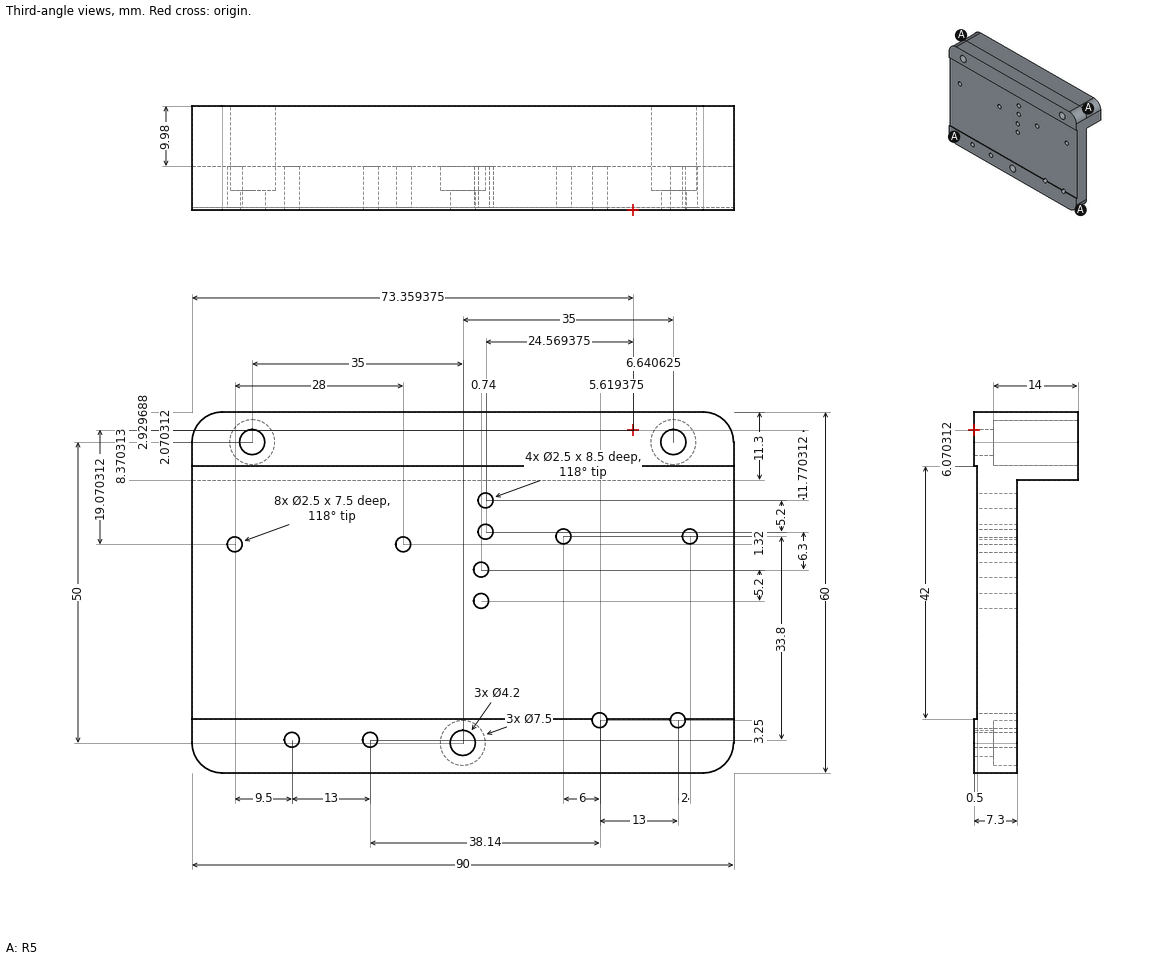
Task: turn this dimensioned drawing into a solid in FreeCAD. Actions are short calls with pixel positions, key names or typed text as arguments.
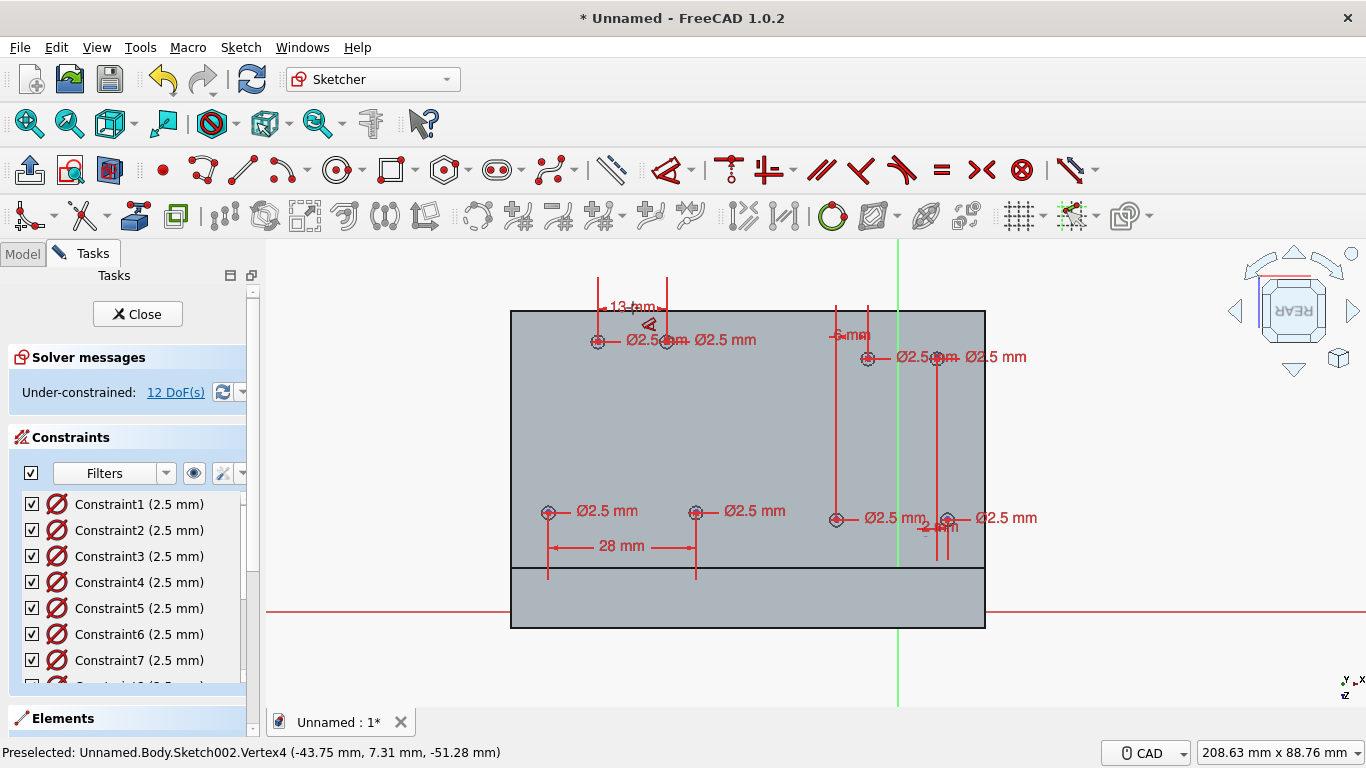
click(868, 359)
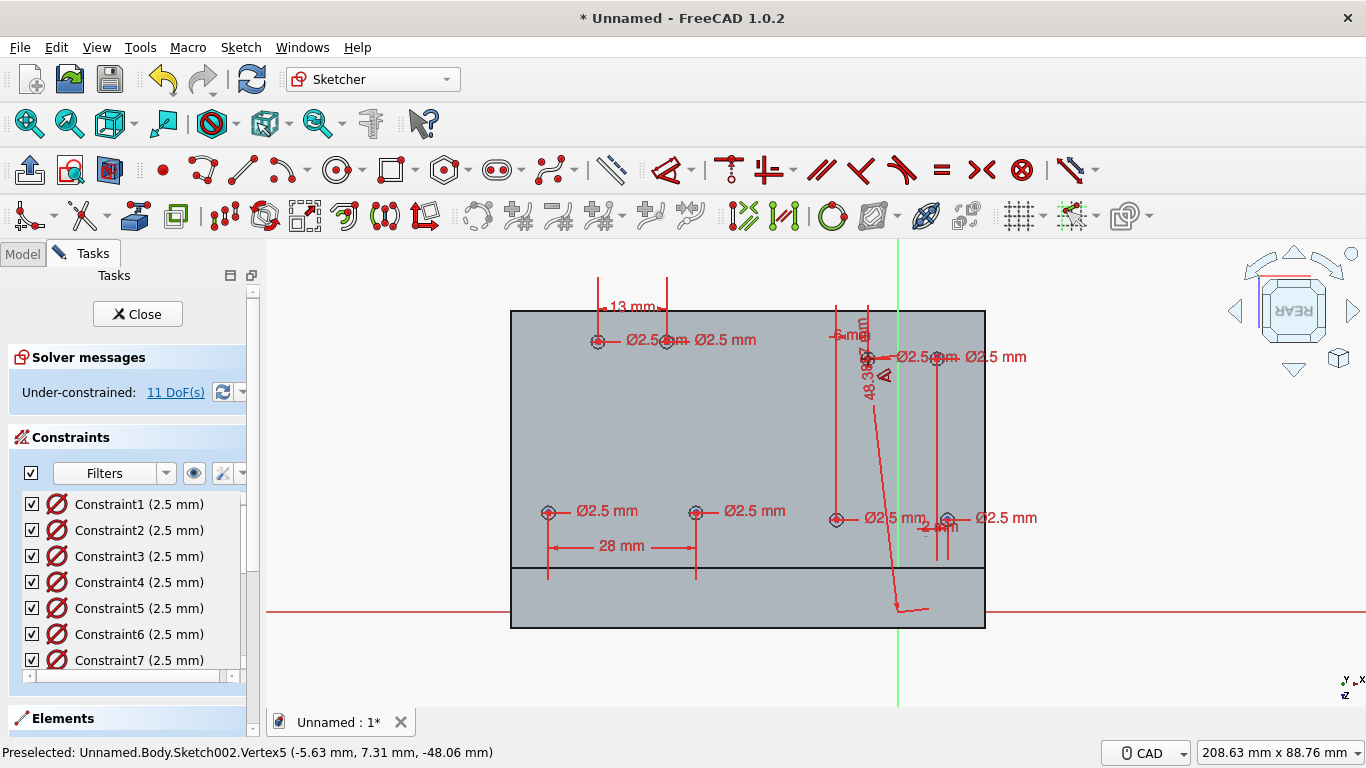
click(937, 359)
click(927, 325)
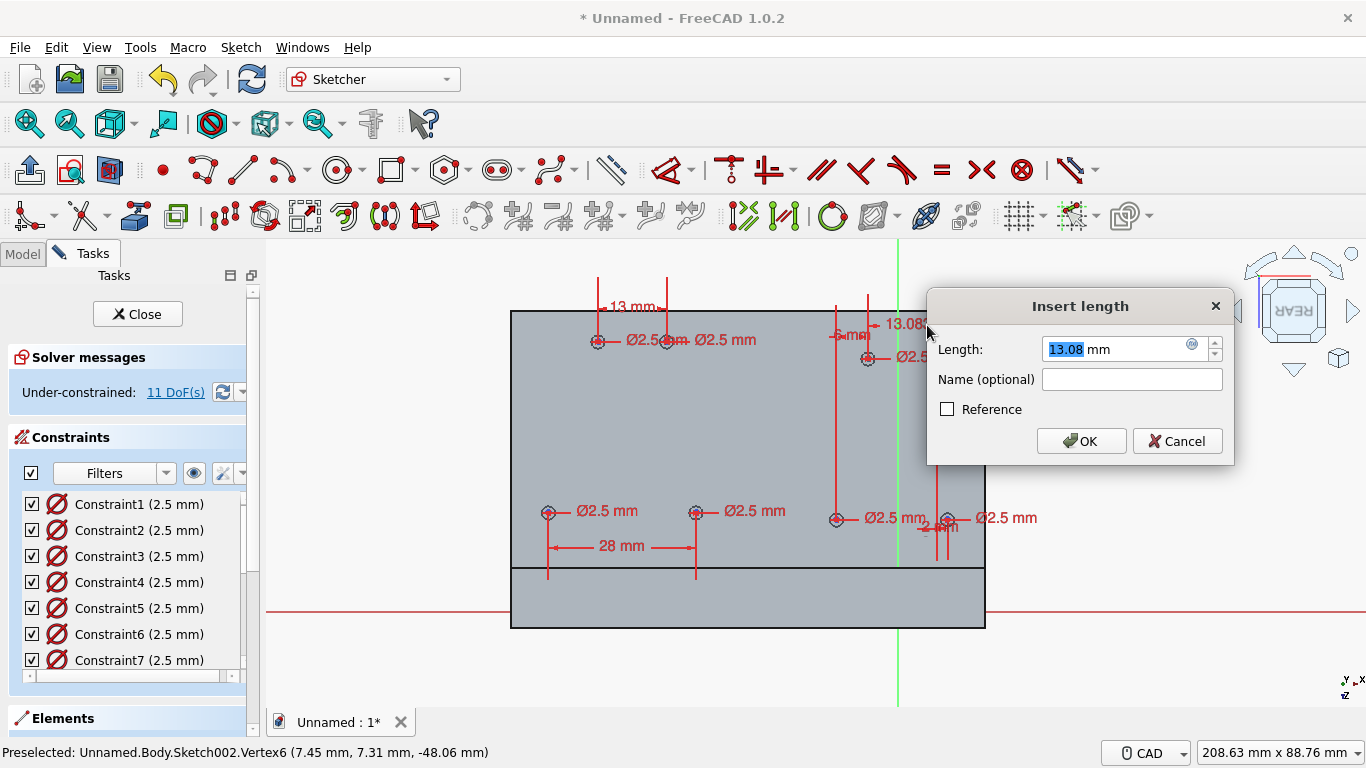
text(13)
key(Return)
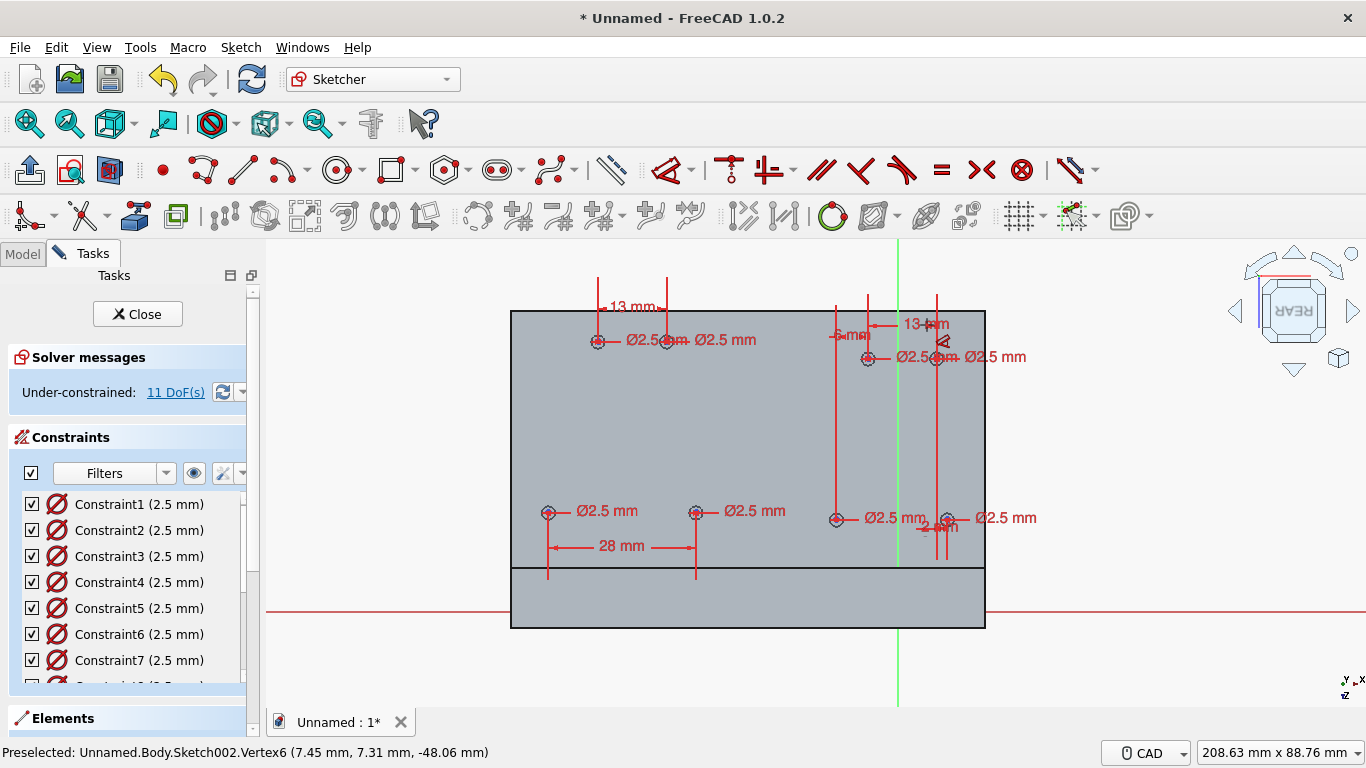
click(548, 513)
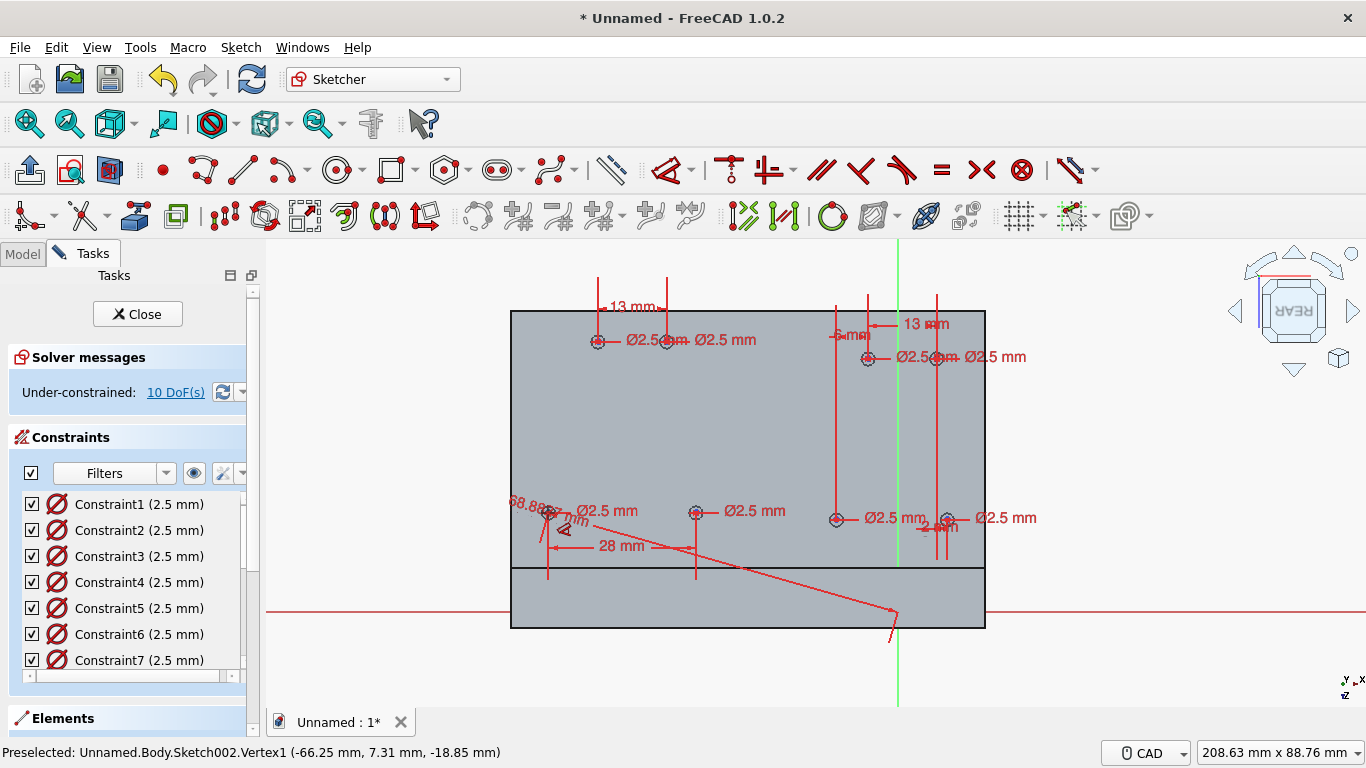
click(598, 342)
click(562, 308)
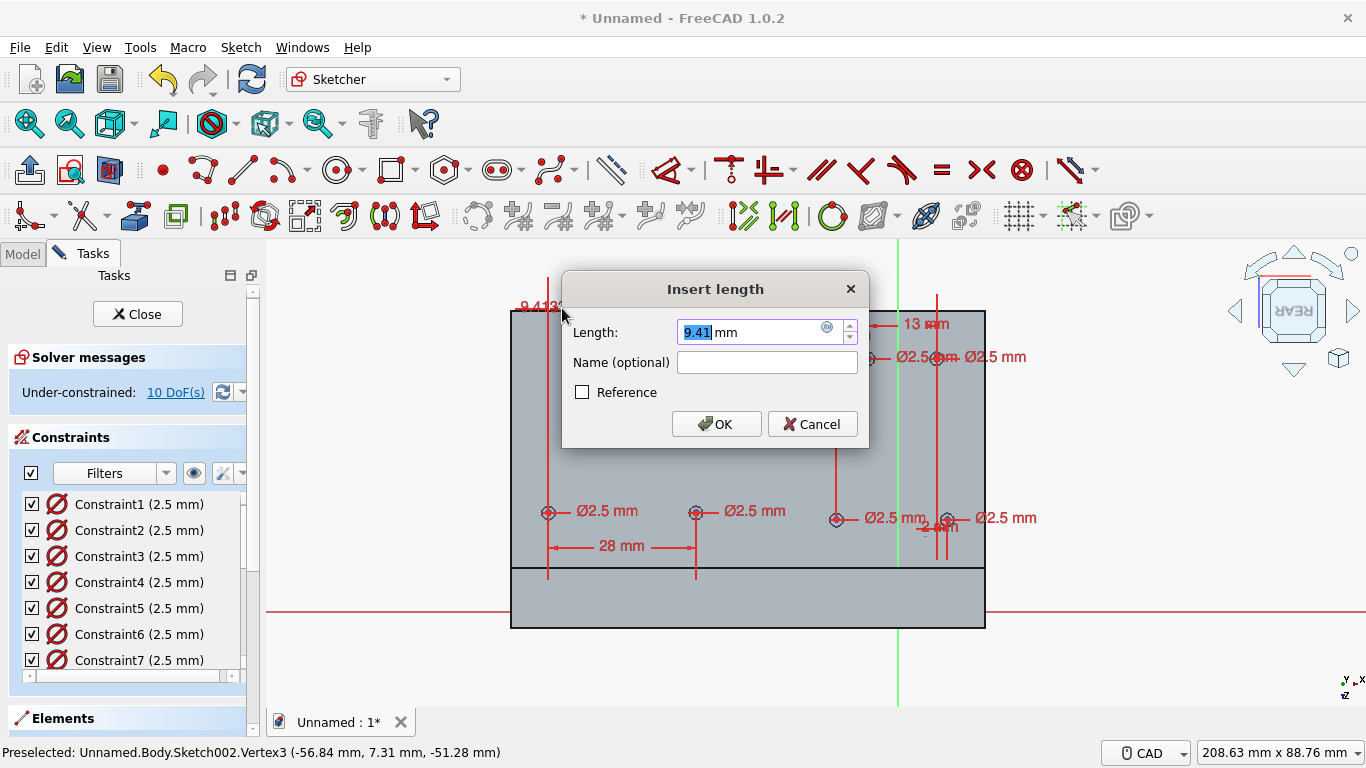
text(9.5)
key(Return)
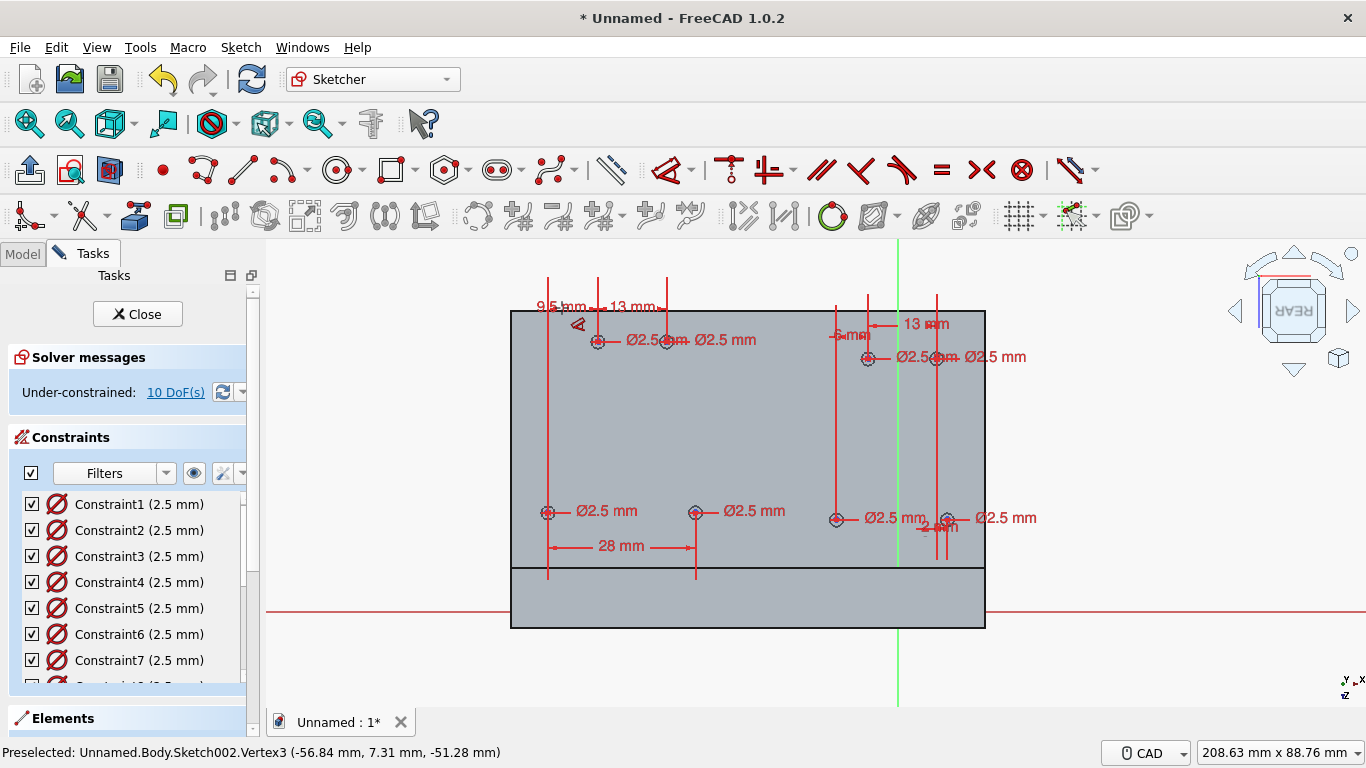
scroll(667, 342, up, 5)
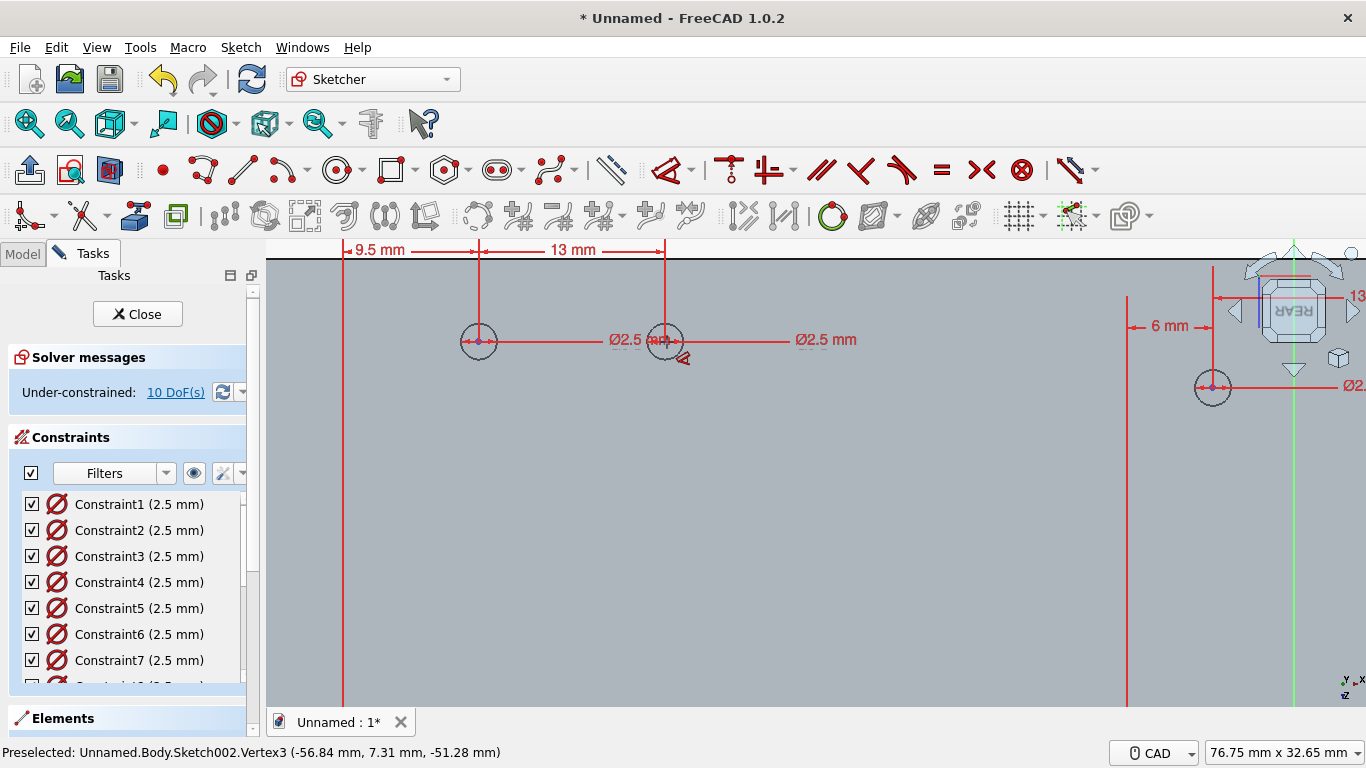
click(665, 342)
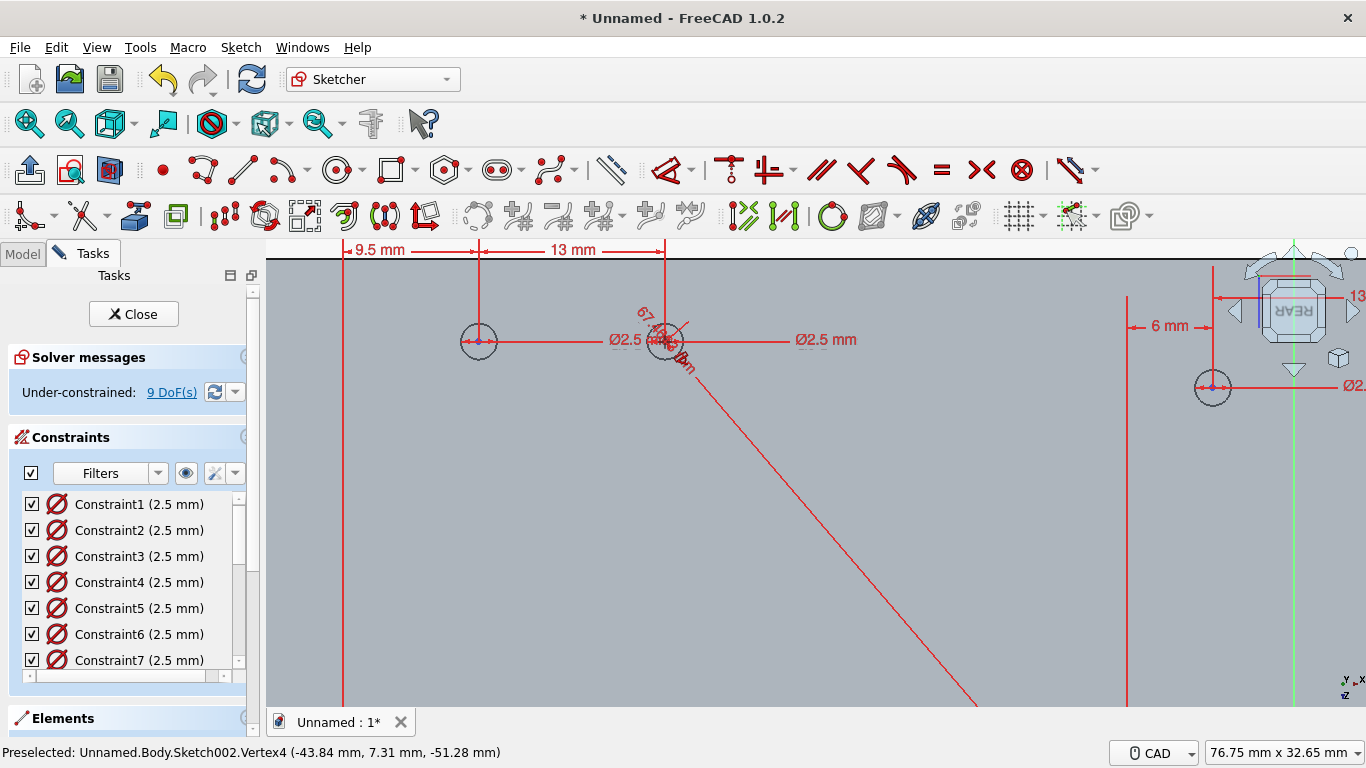
scroll(667, 342, down, 5)